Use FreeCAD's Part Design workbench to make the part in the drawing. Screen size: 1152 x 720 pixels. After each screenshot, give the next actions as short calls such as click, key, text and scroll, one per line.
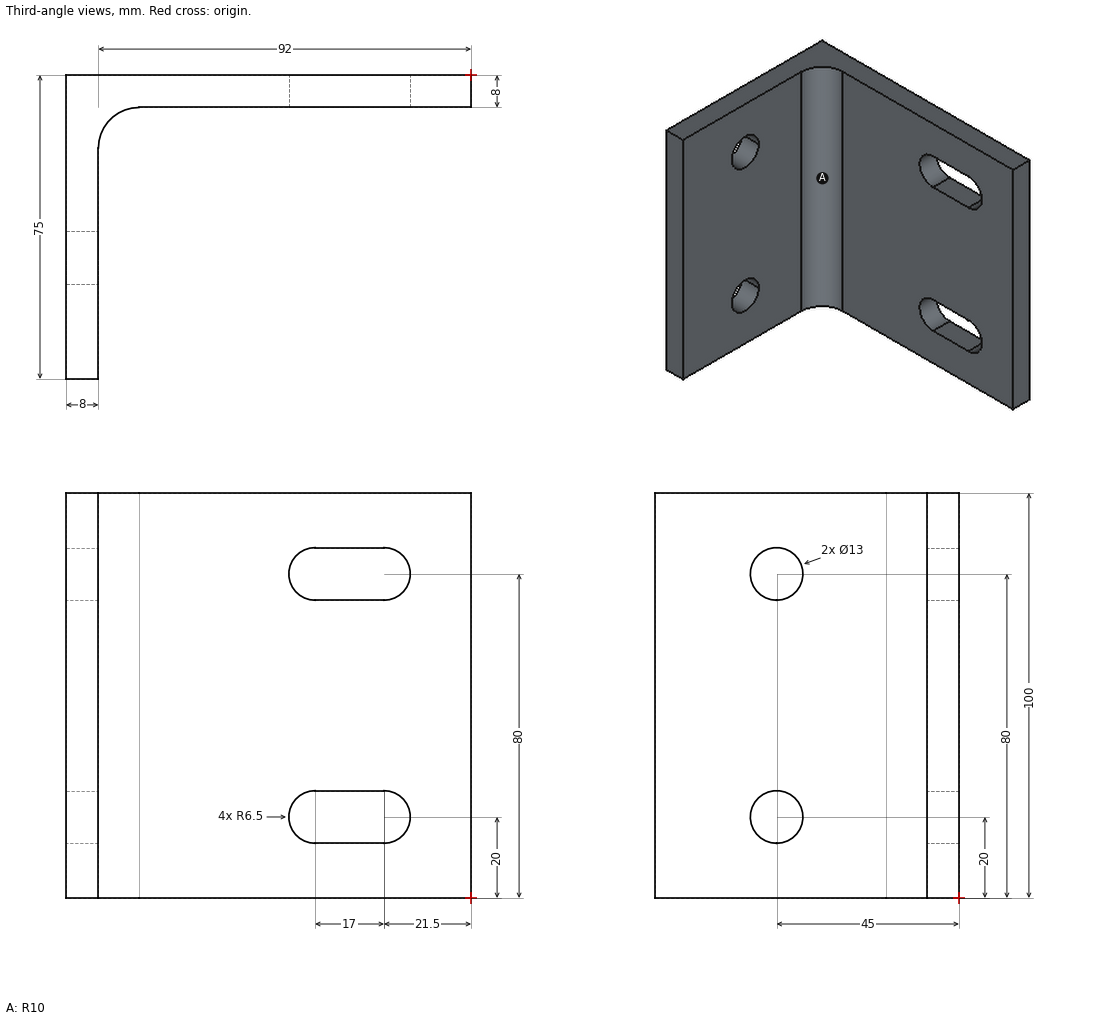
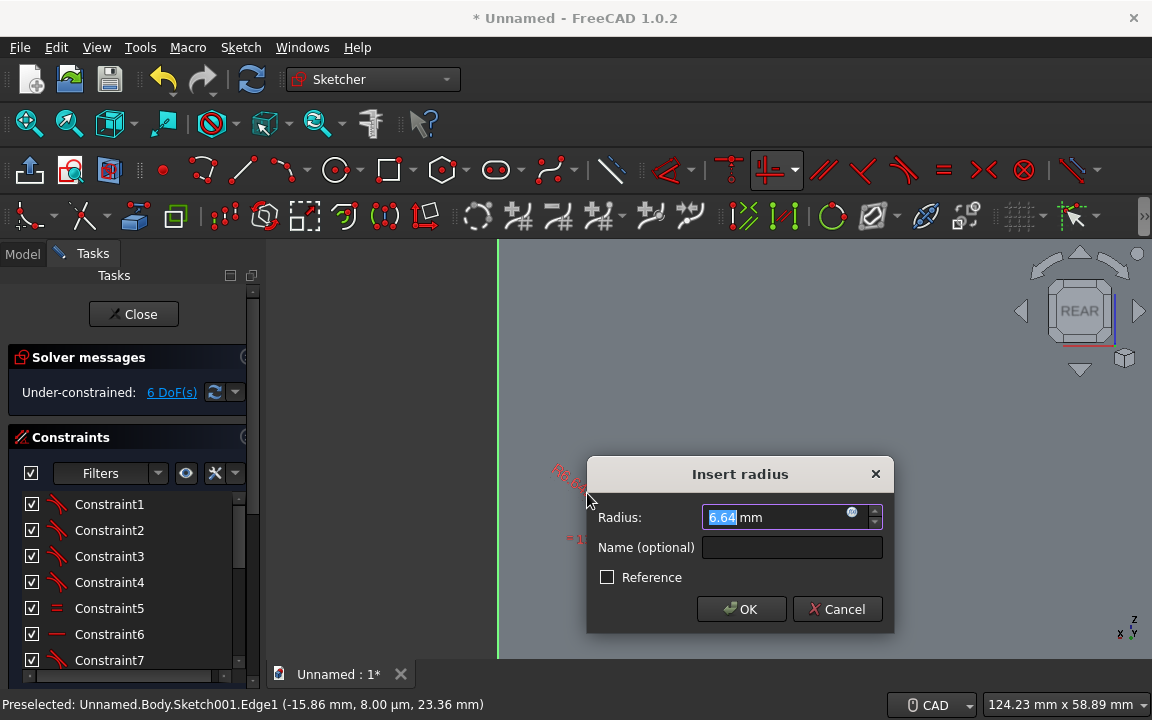
text(6.5)
key(Return)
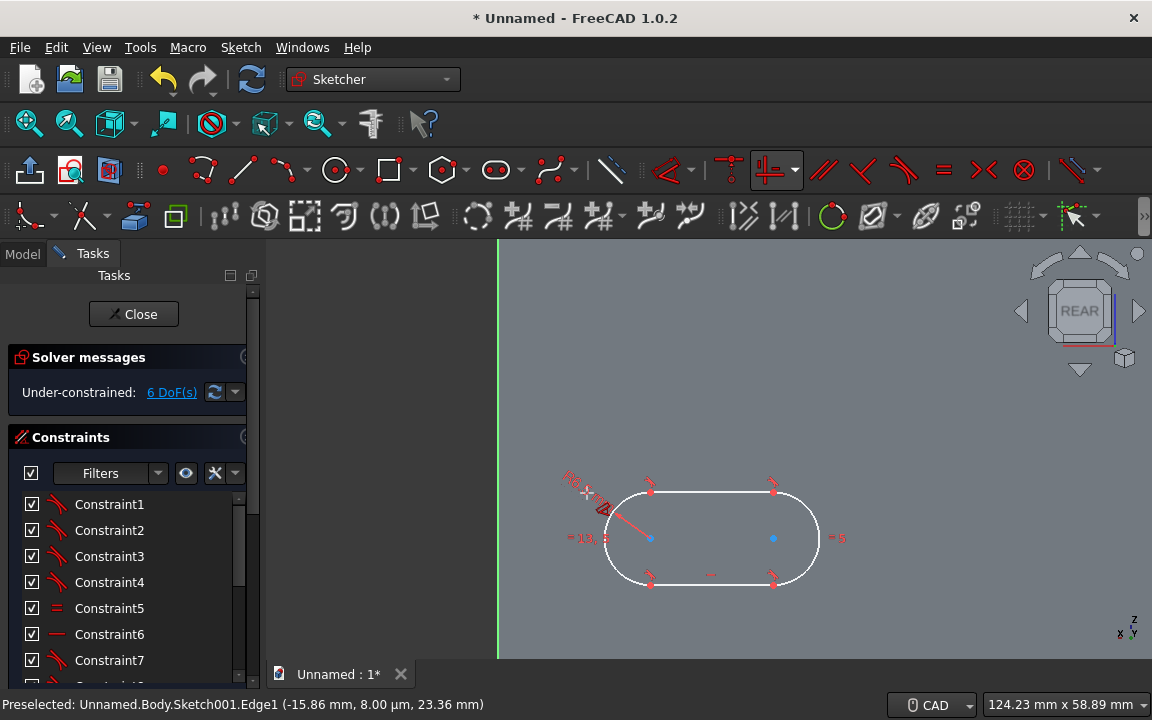
click(688, 492)
click(712, 526)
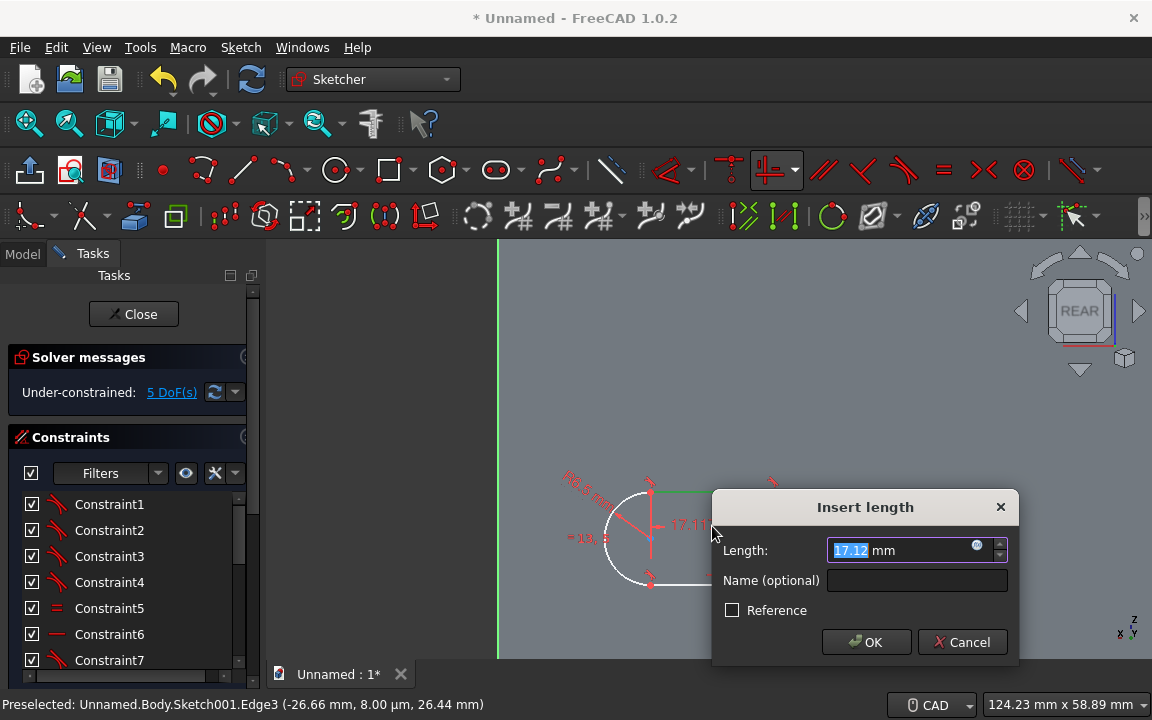
text(17)
key(Return)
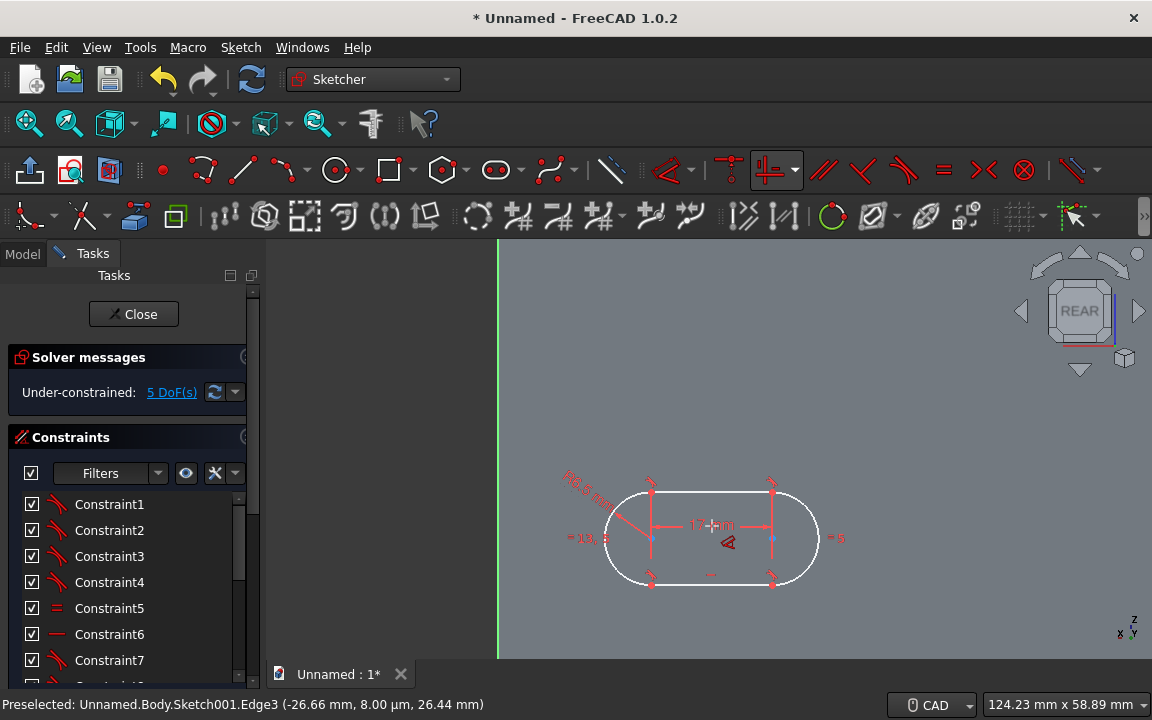
scroll(626, 511, down, 4)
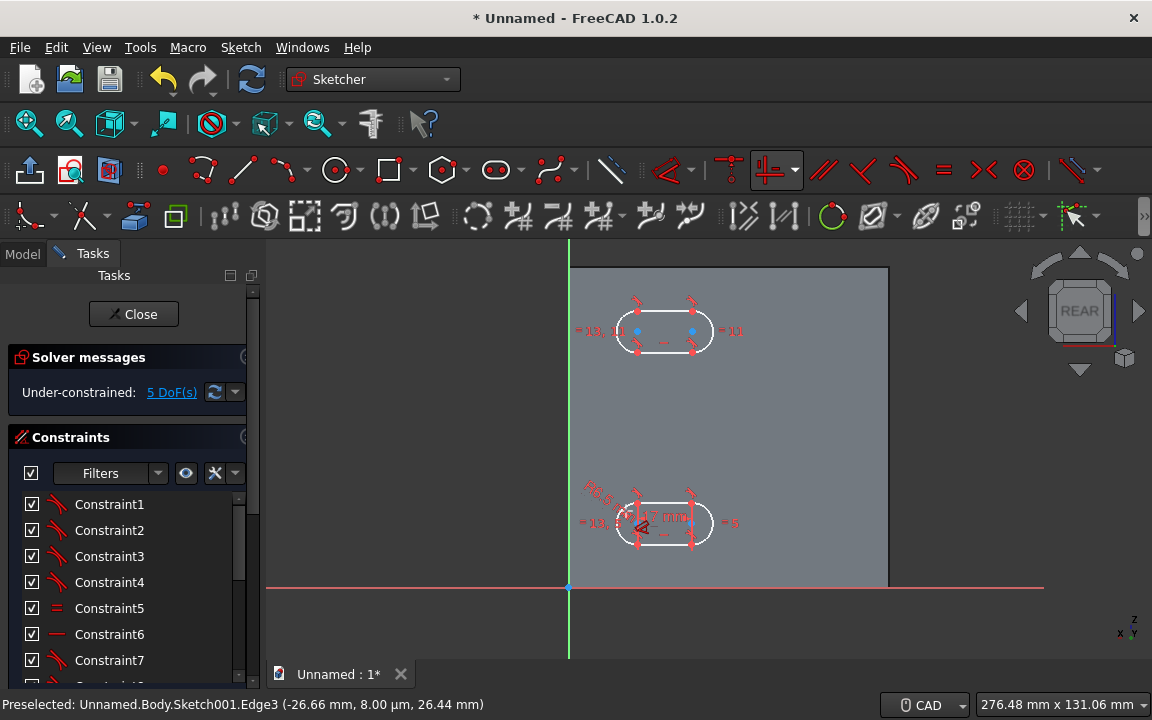
click(654, 311)
click(665, 277)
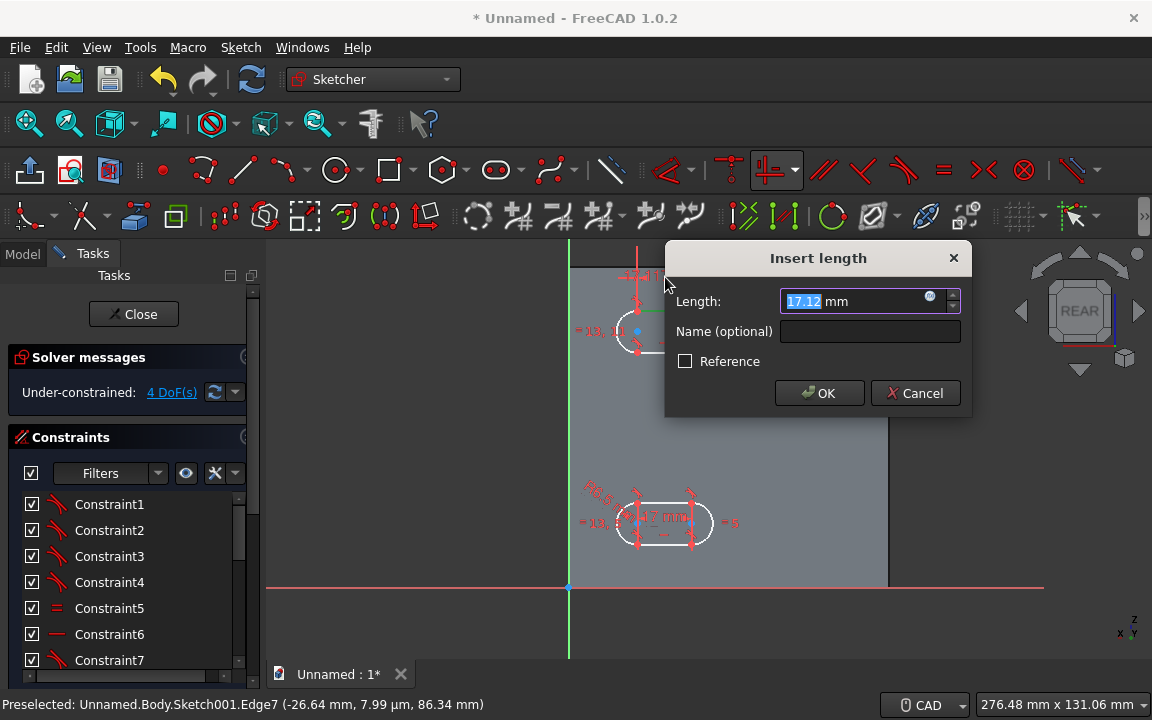
text(17)
key(Return)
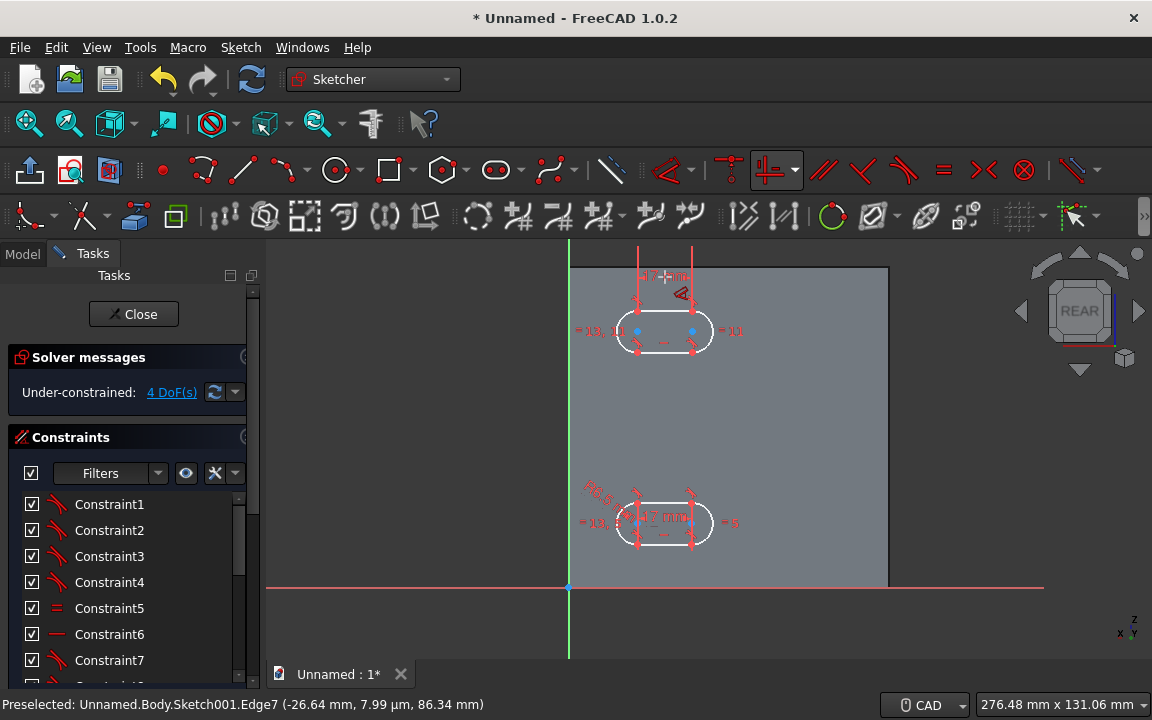
click(638, 524)
click(535, 556)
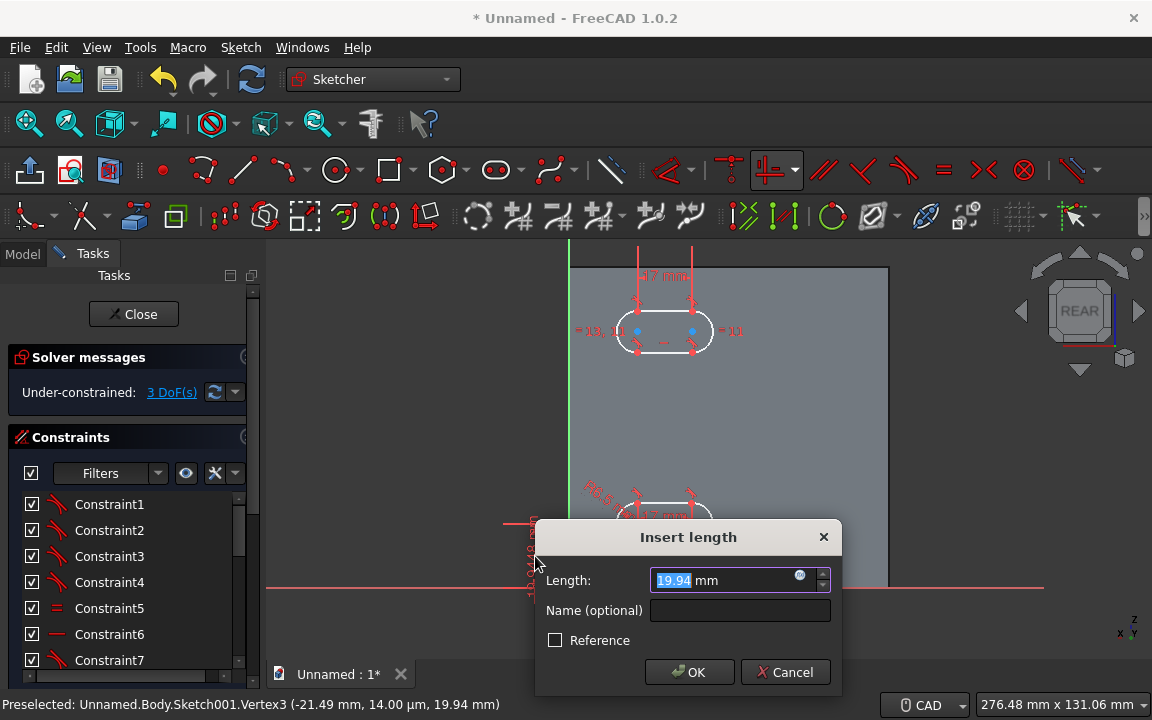
text(20)
key(Return)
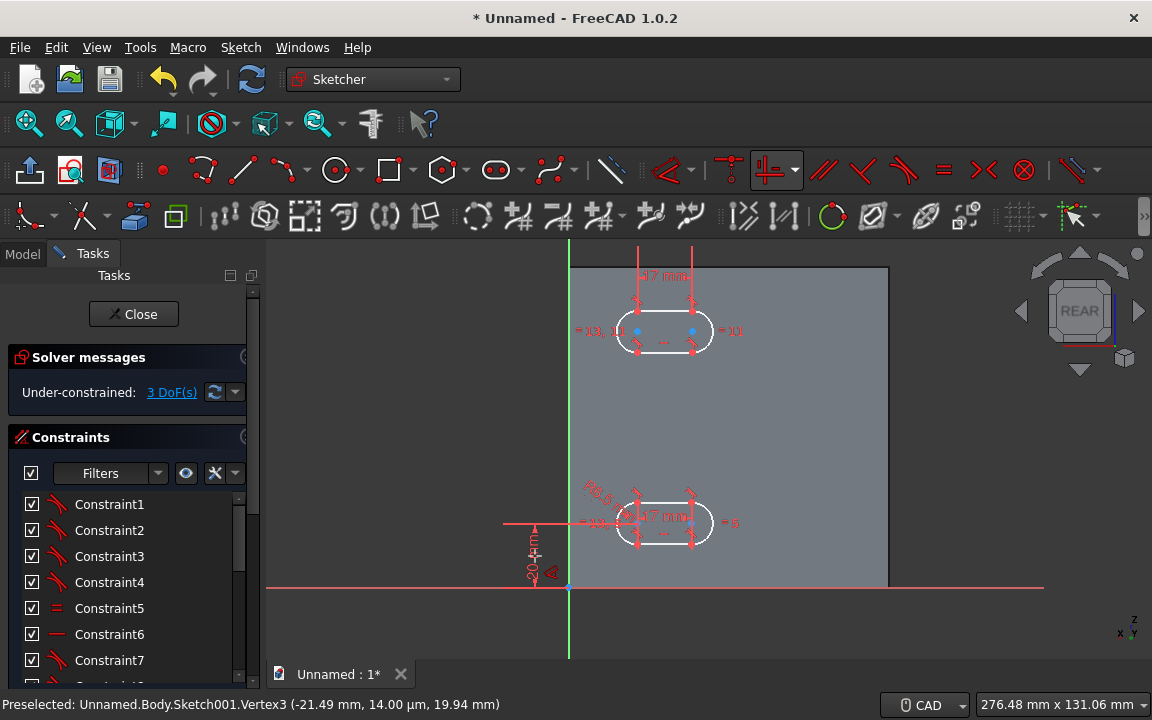
click(638, 332)
click(535, 460)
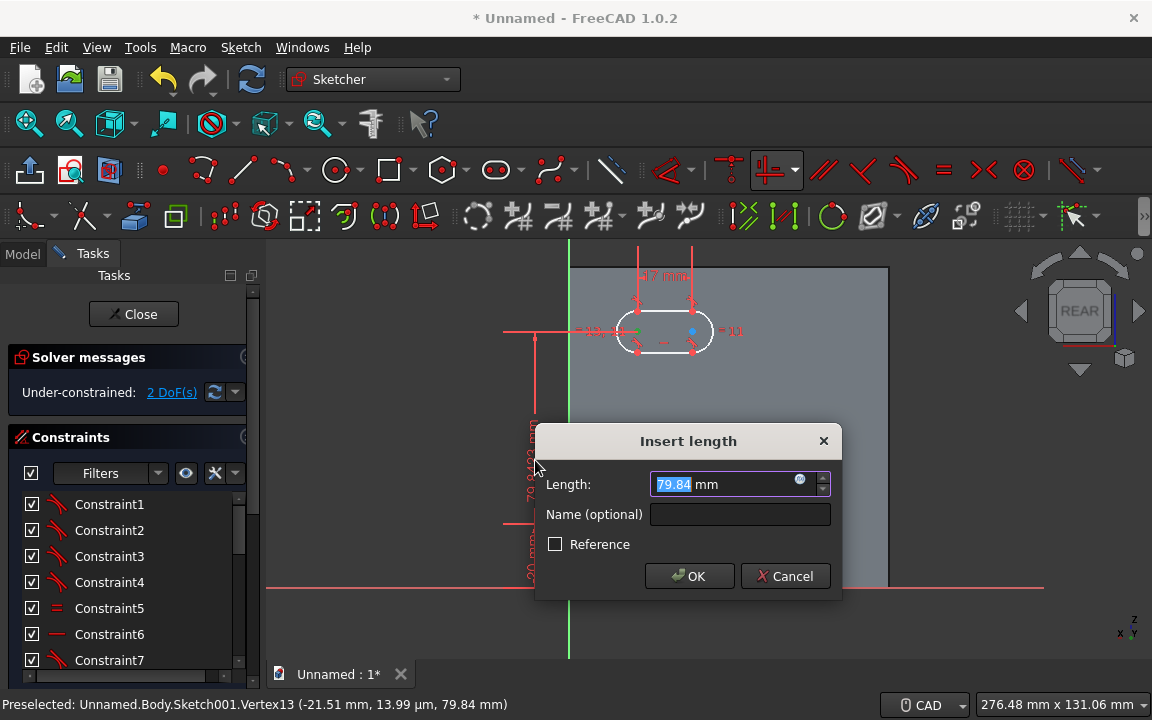
text(80)
key(Return)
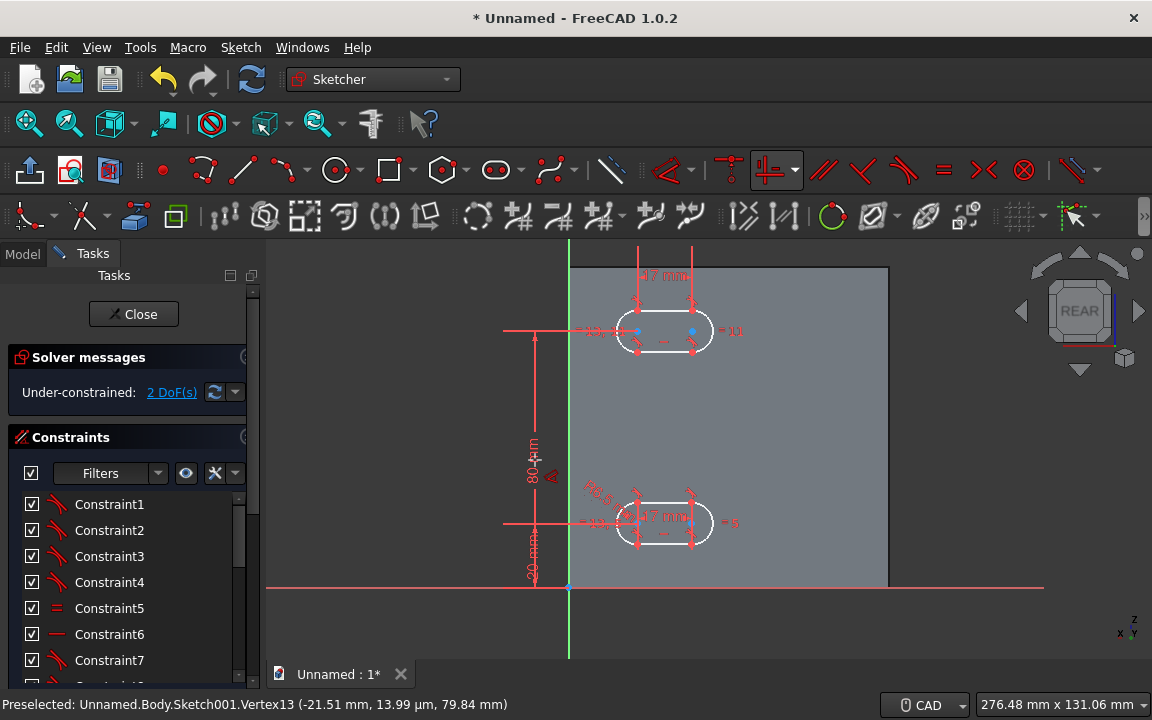
click(638, 503)
click(603, 622)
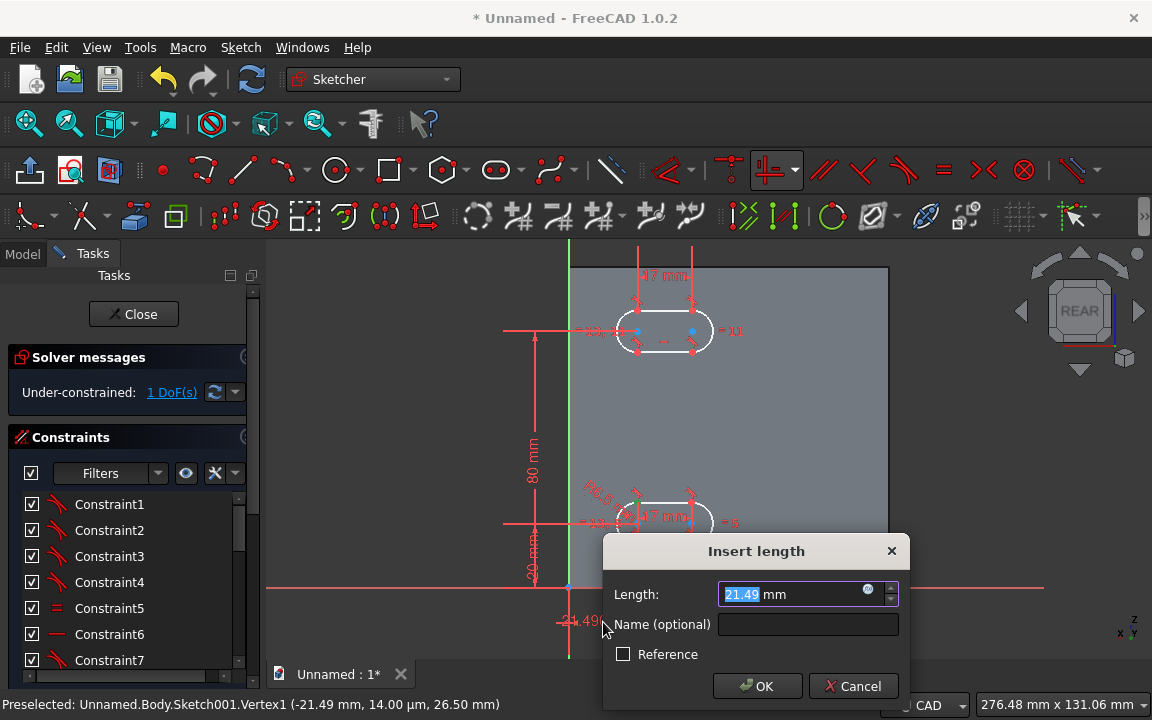
text(21.5)
key(Return)